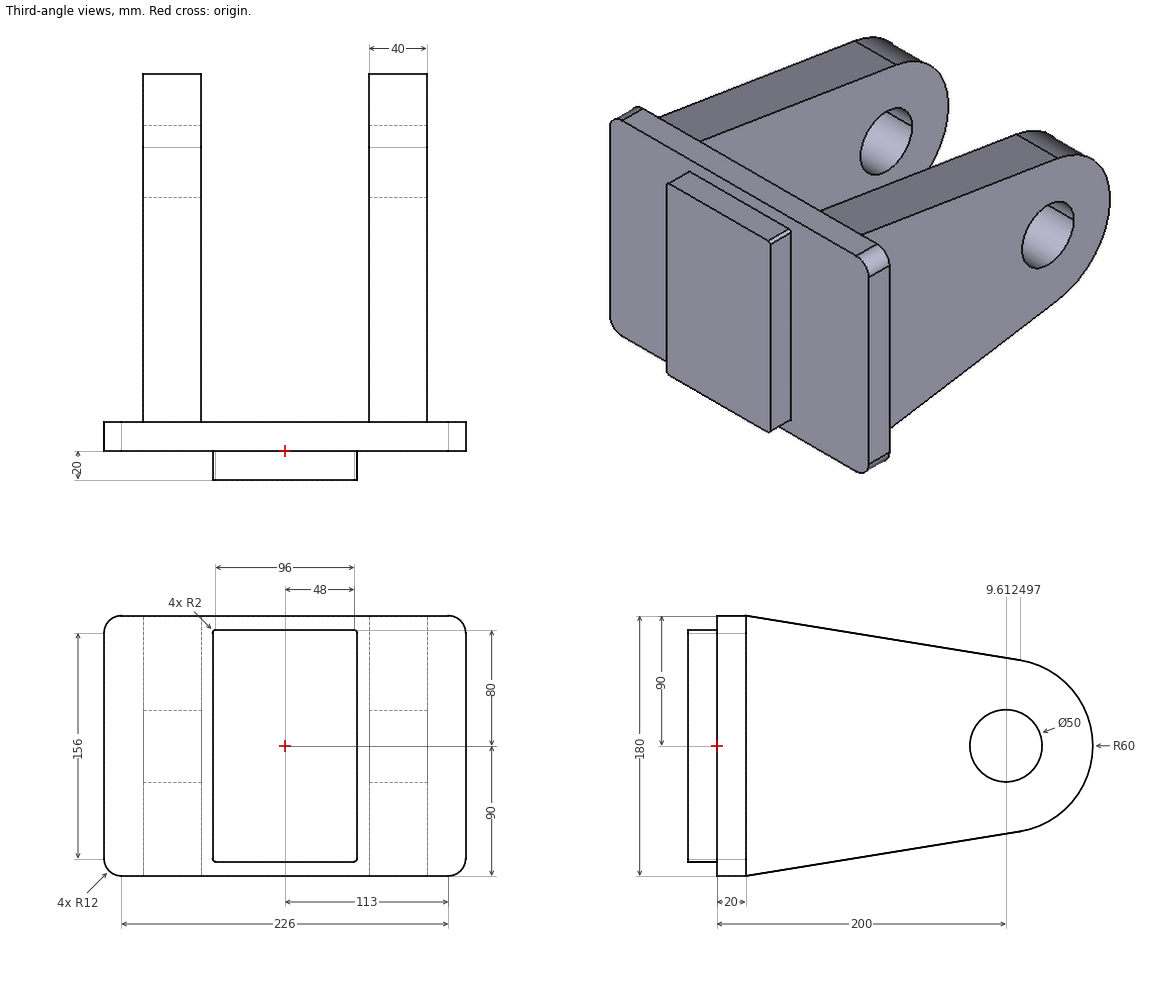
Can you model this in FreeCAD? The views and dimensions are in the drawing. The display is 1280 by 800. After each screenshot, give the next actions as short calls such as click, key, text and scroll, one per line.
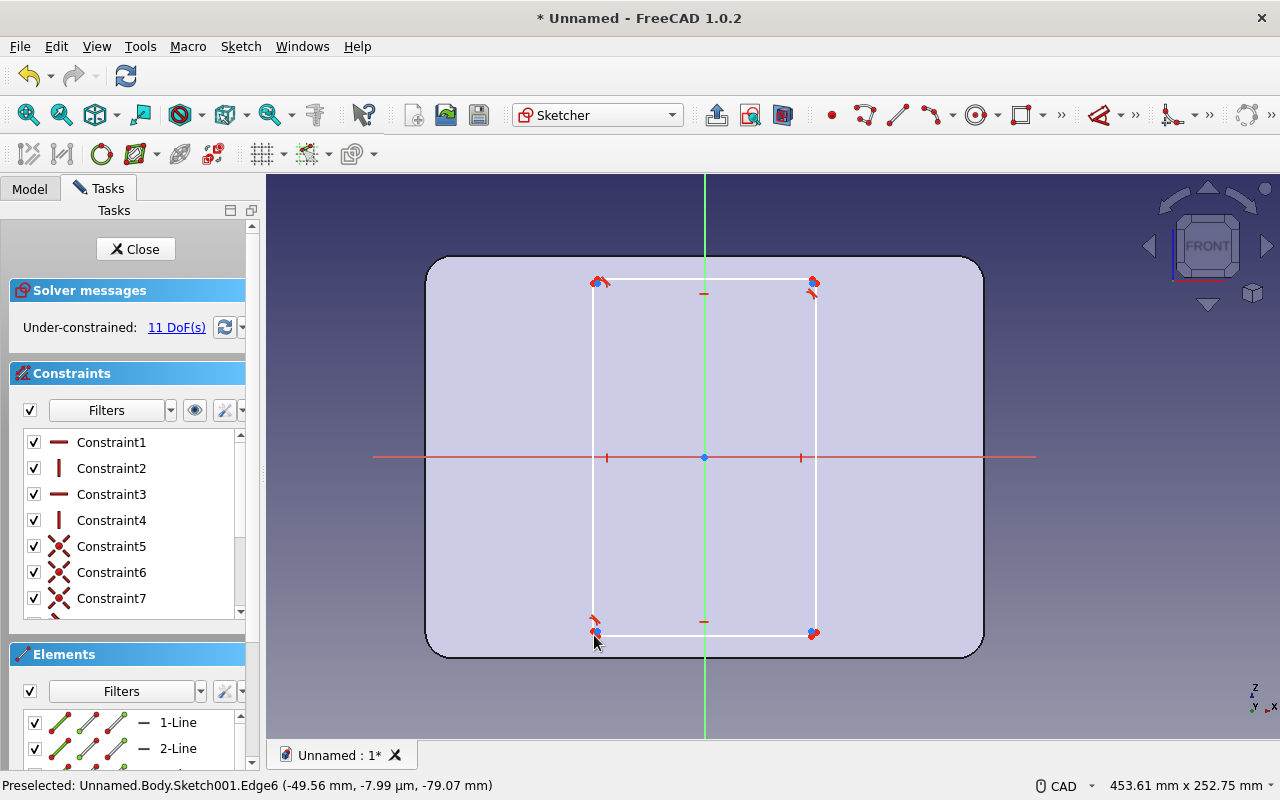
click(662, 636)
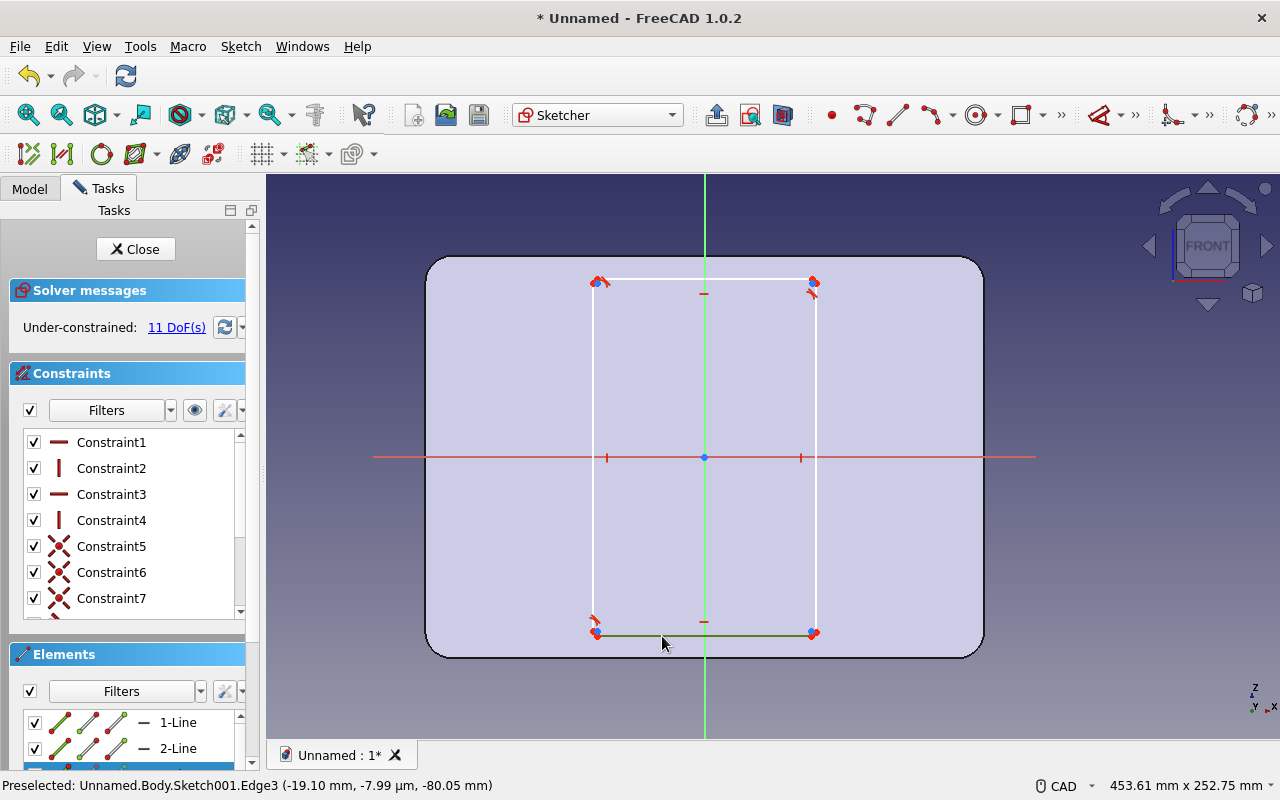
scroll(815, 635, up, 8)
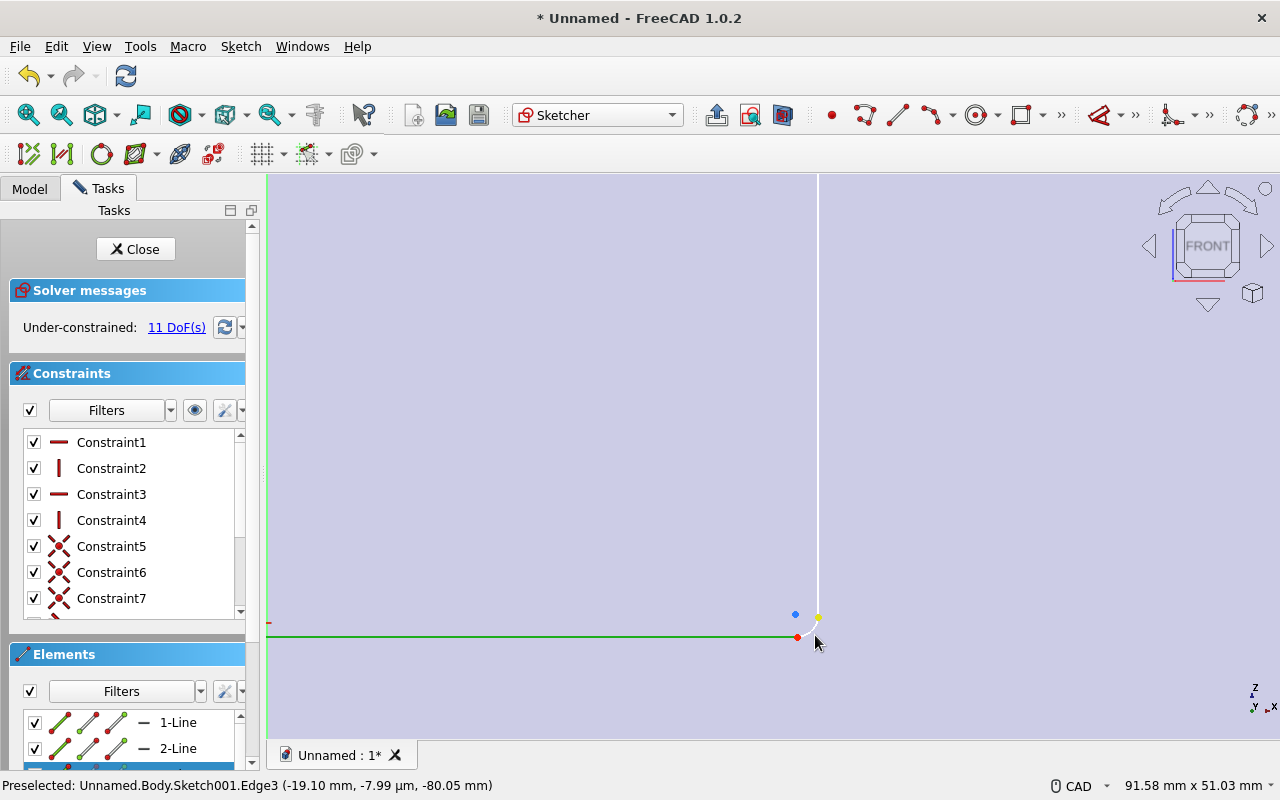
click(812, 631)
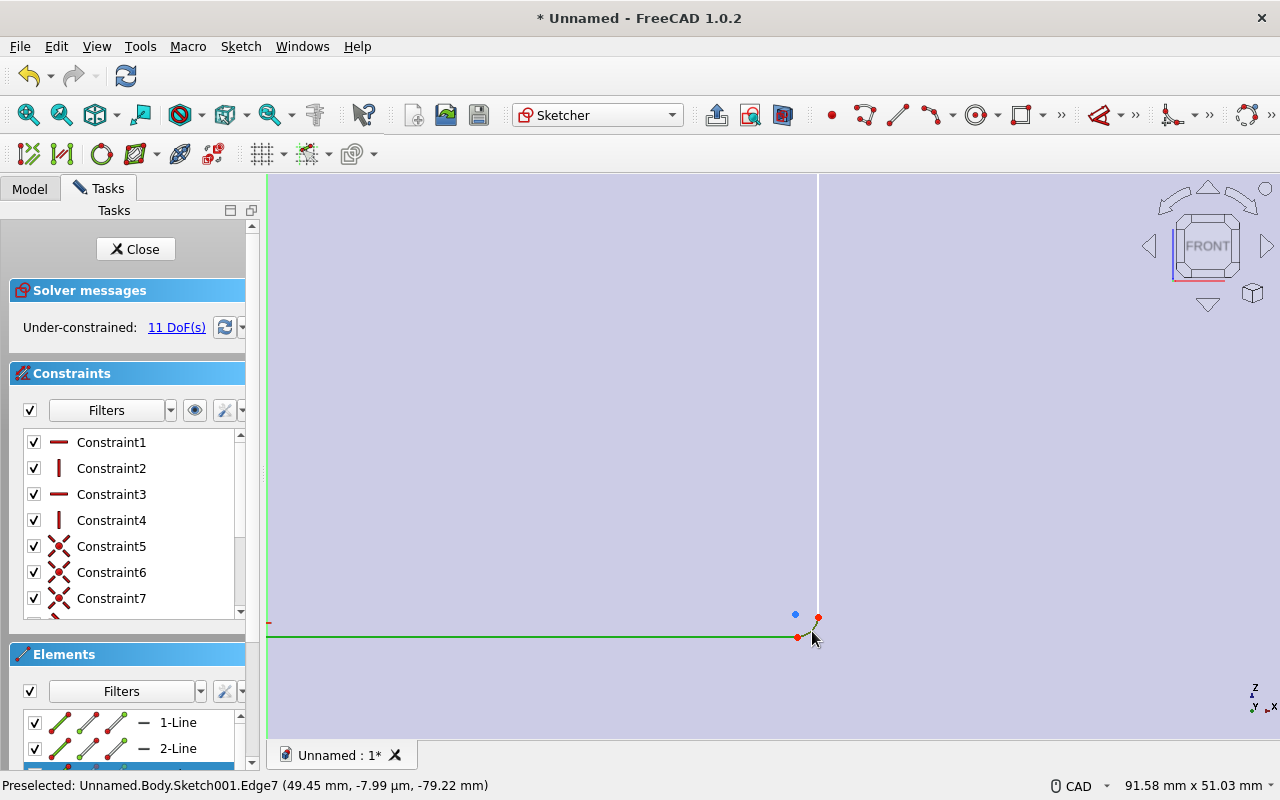
key(t)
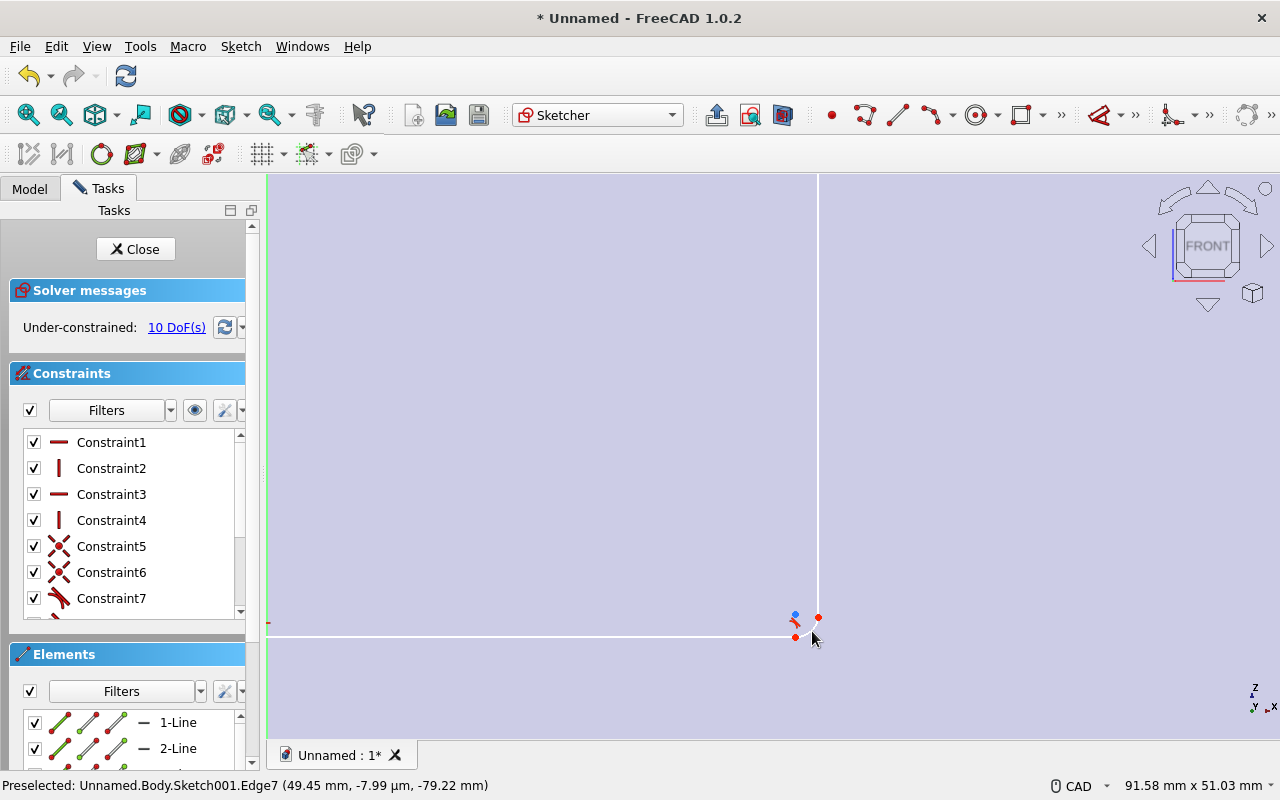
scroll(815, 635, down, 8)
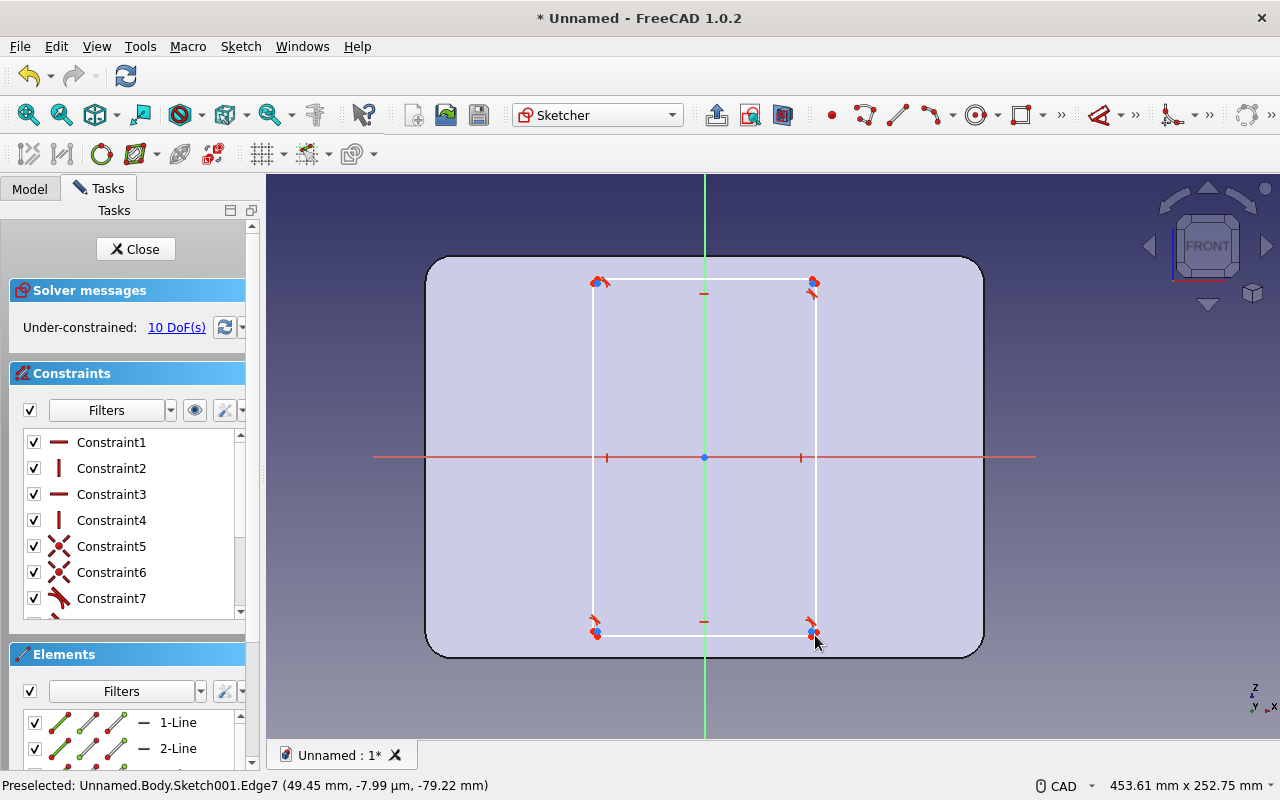
click(816, 562)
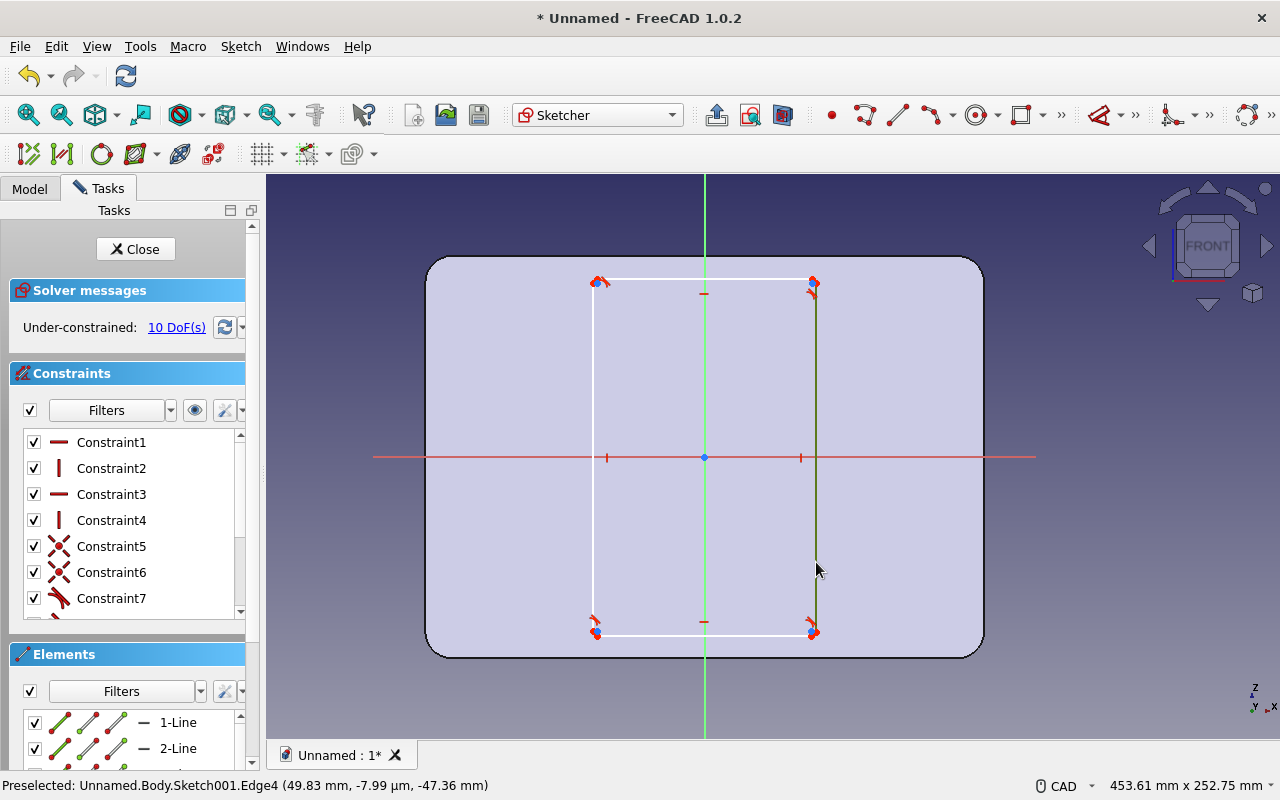
scroll(815, 635, up, 8)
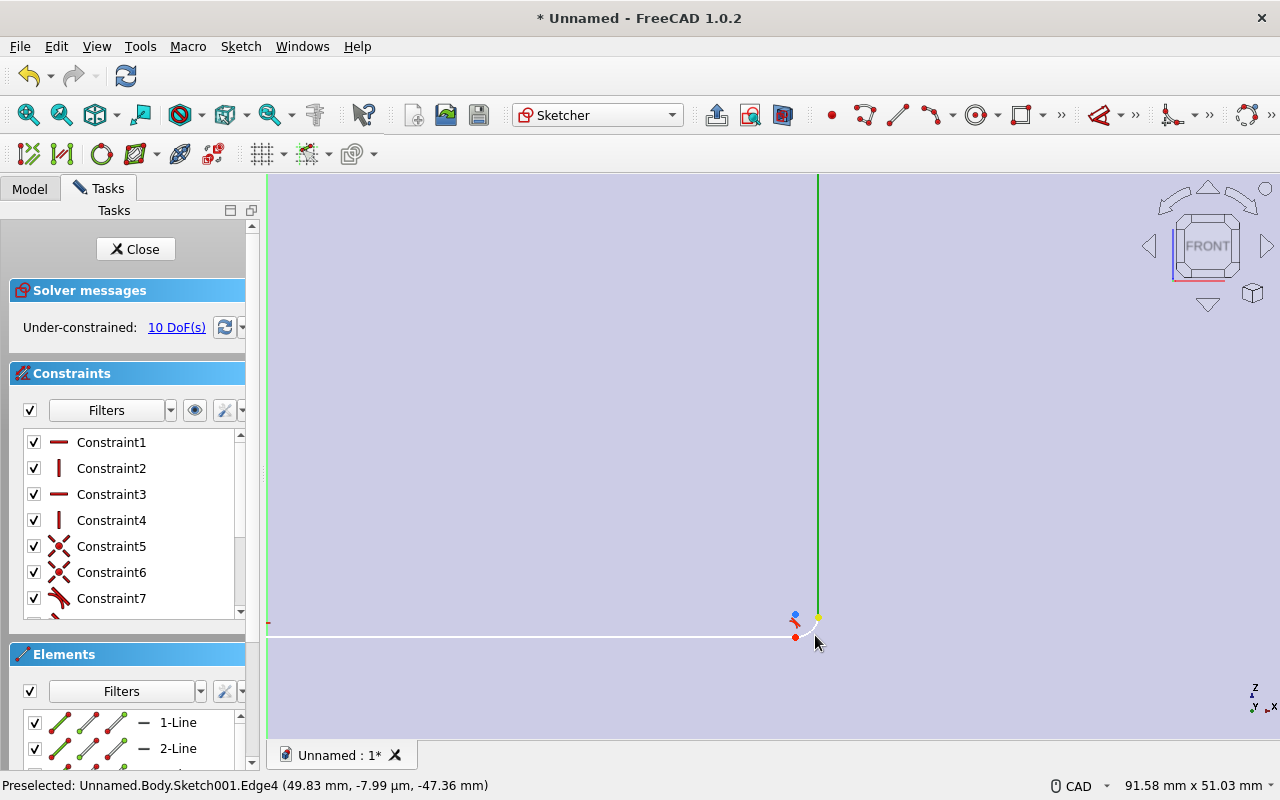
click(811, 631)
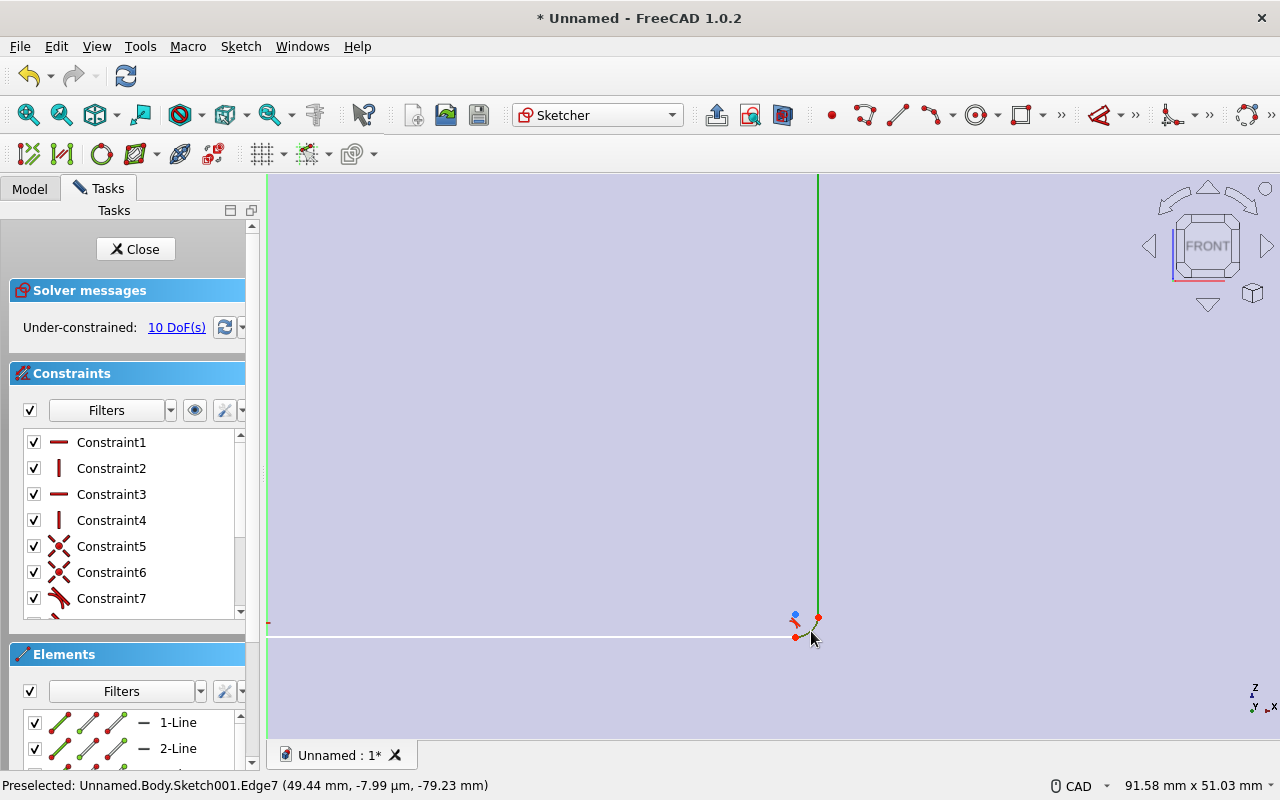
key(t)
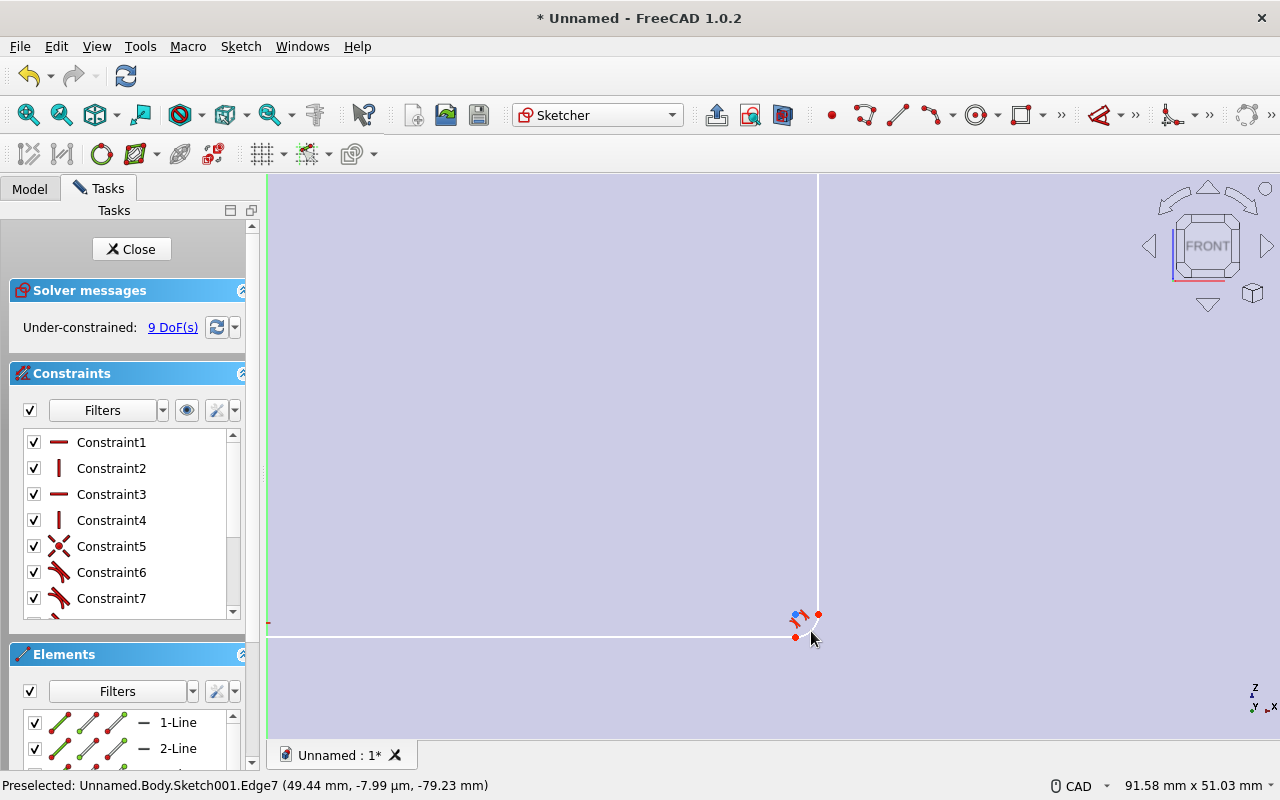
scroll(815, 635, down, 8)